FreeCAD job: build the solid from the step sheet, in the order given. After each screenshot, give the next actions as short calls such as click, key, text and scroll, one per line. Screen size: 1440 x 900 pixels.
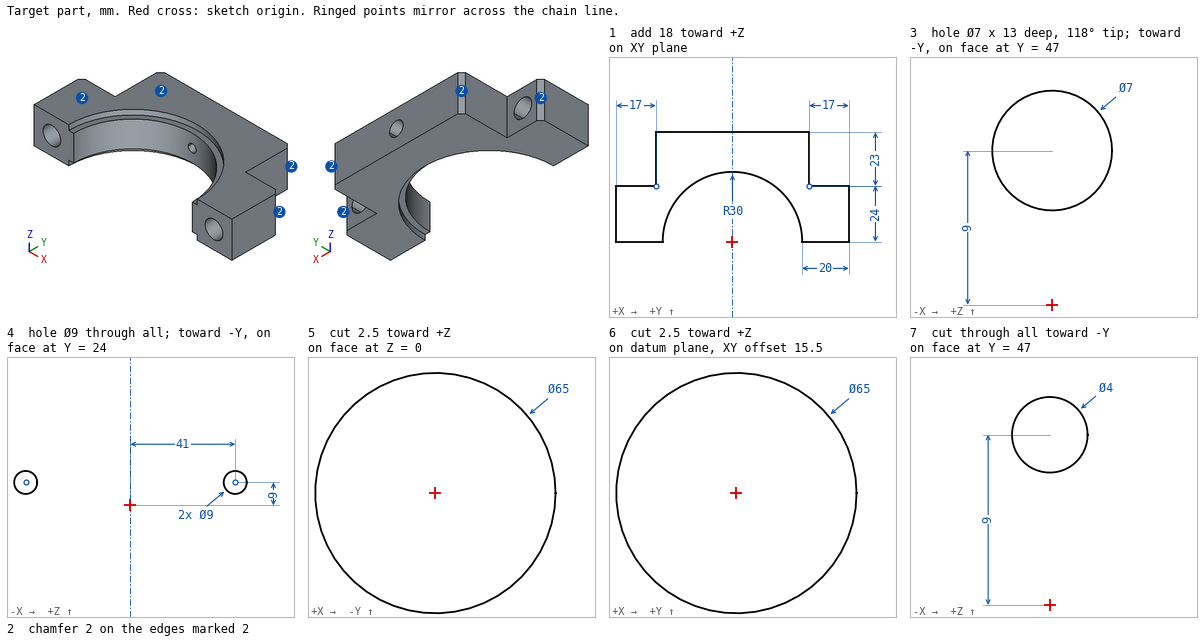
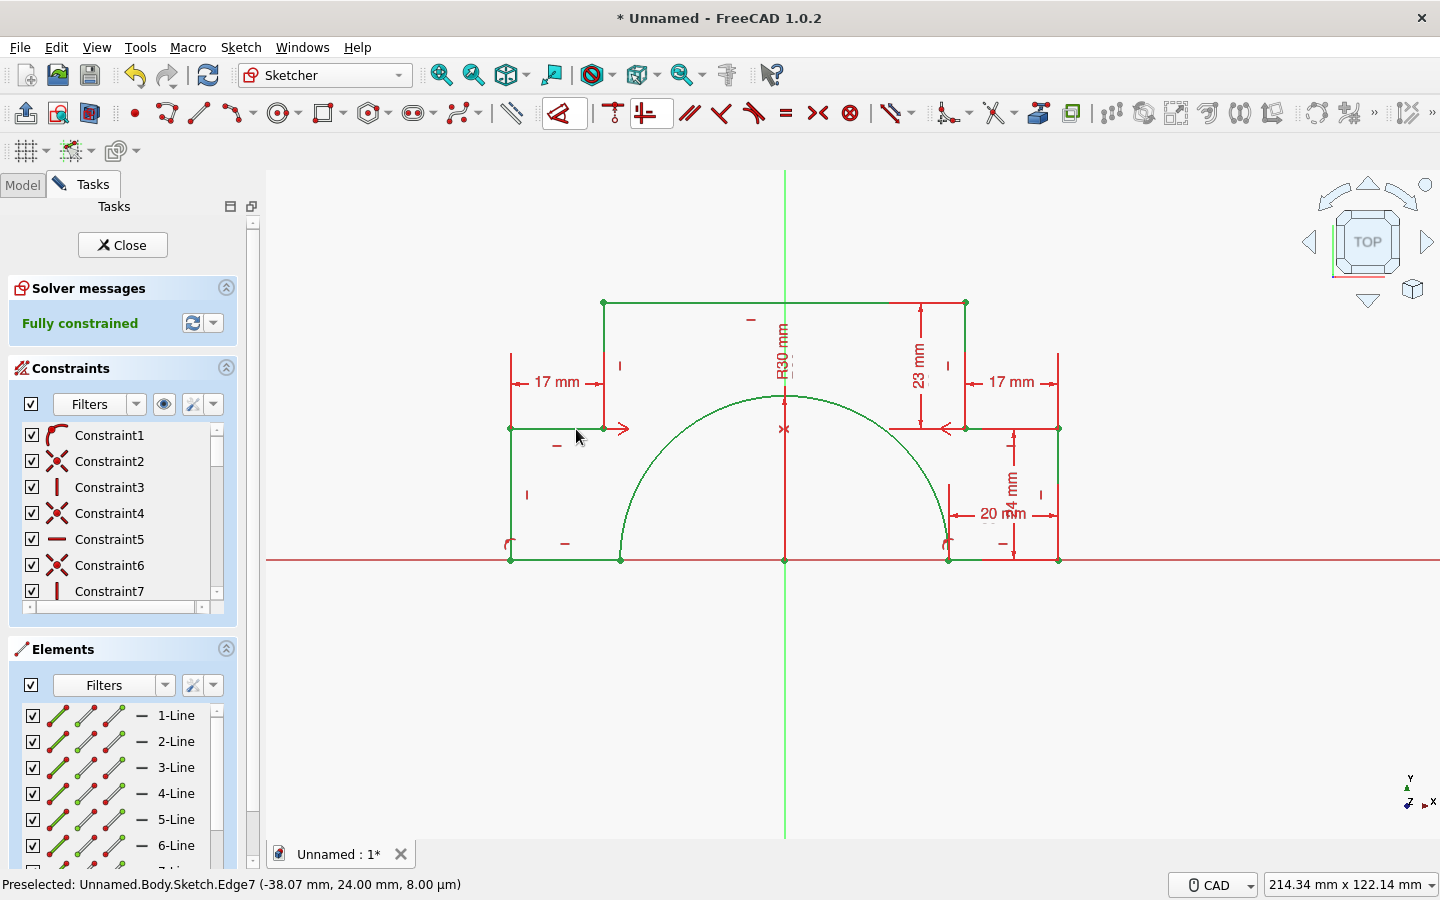
click(123, 245)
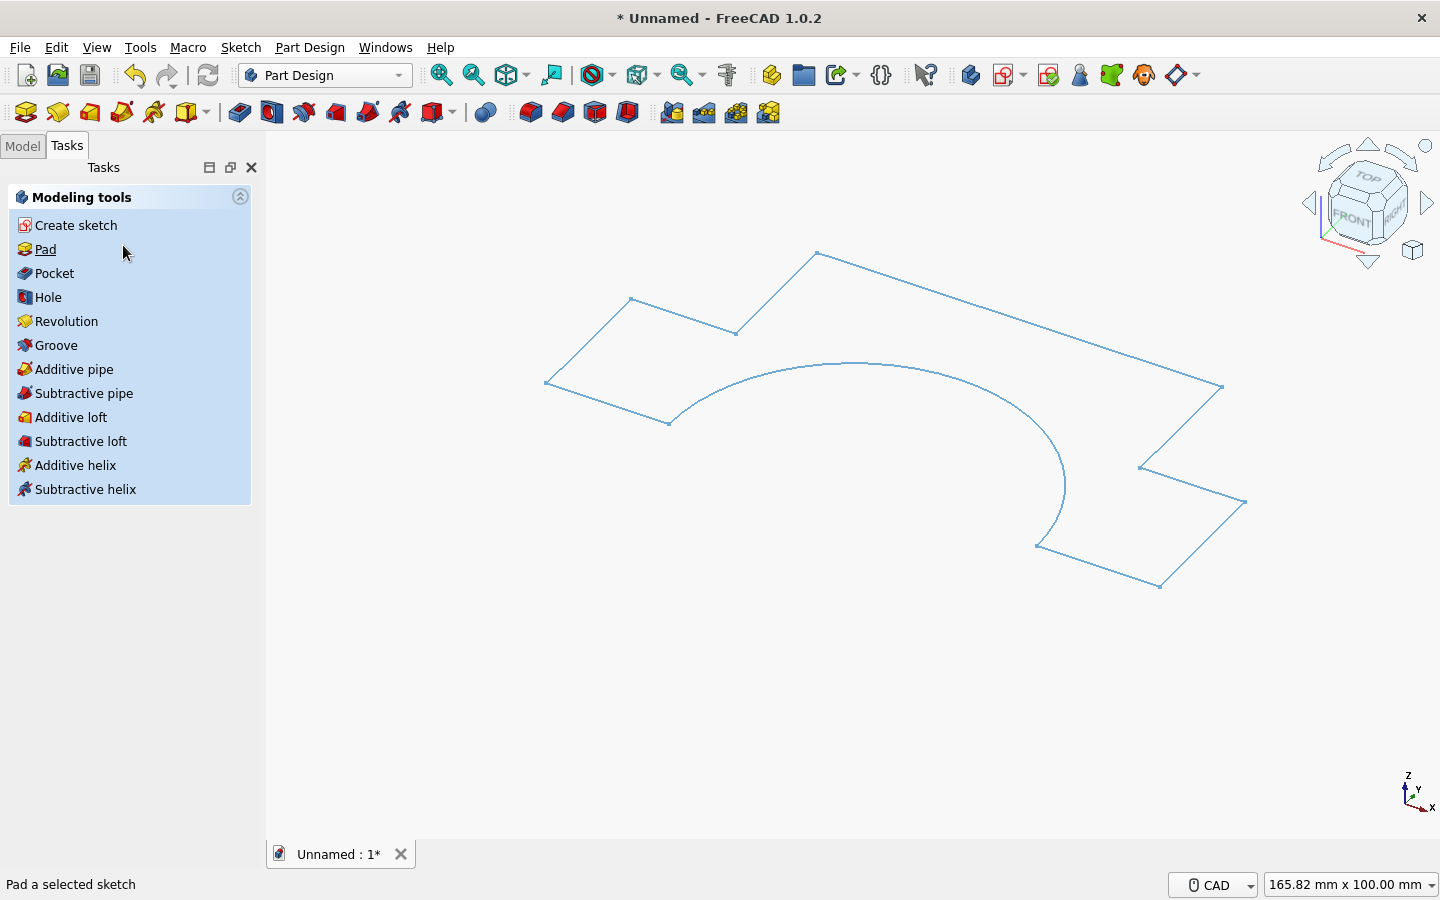
click(26, 112)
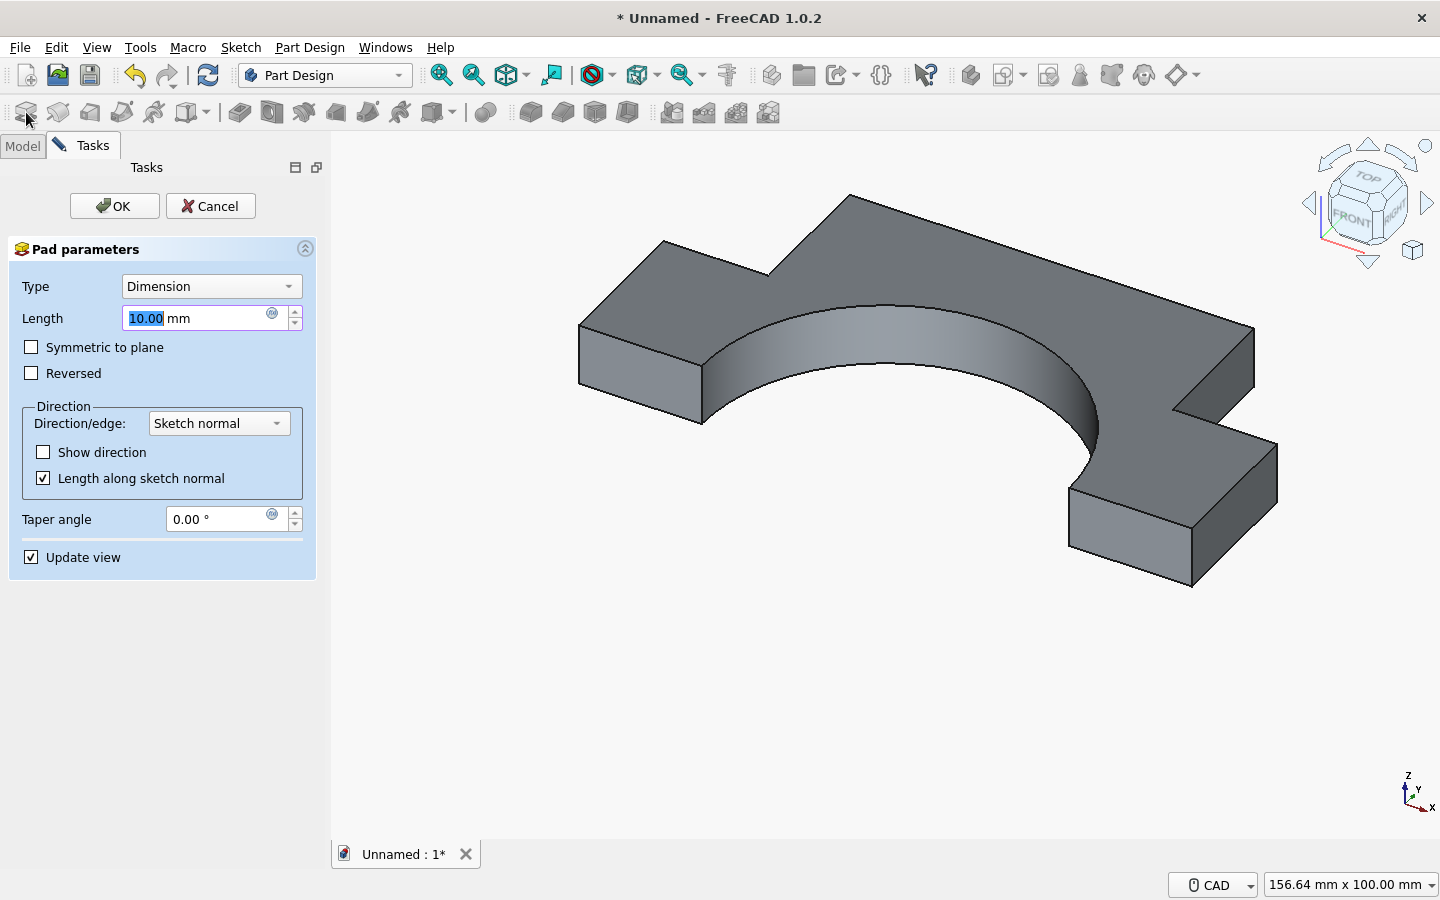
text(18)
key(Tab)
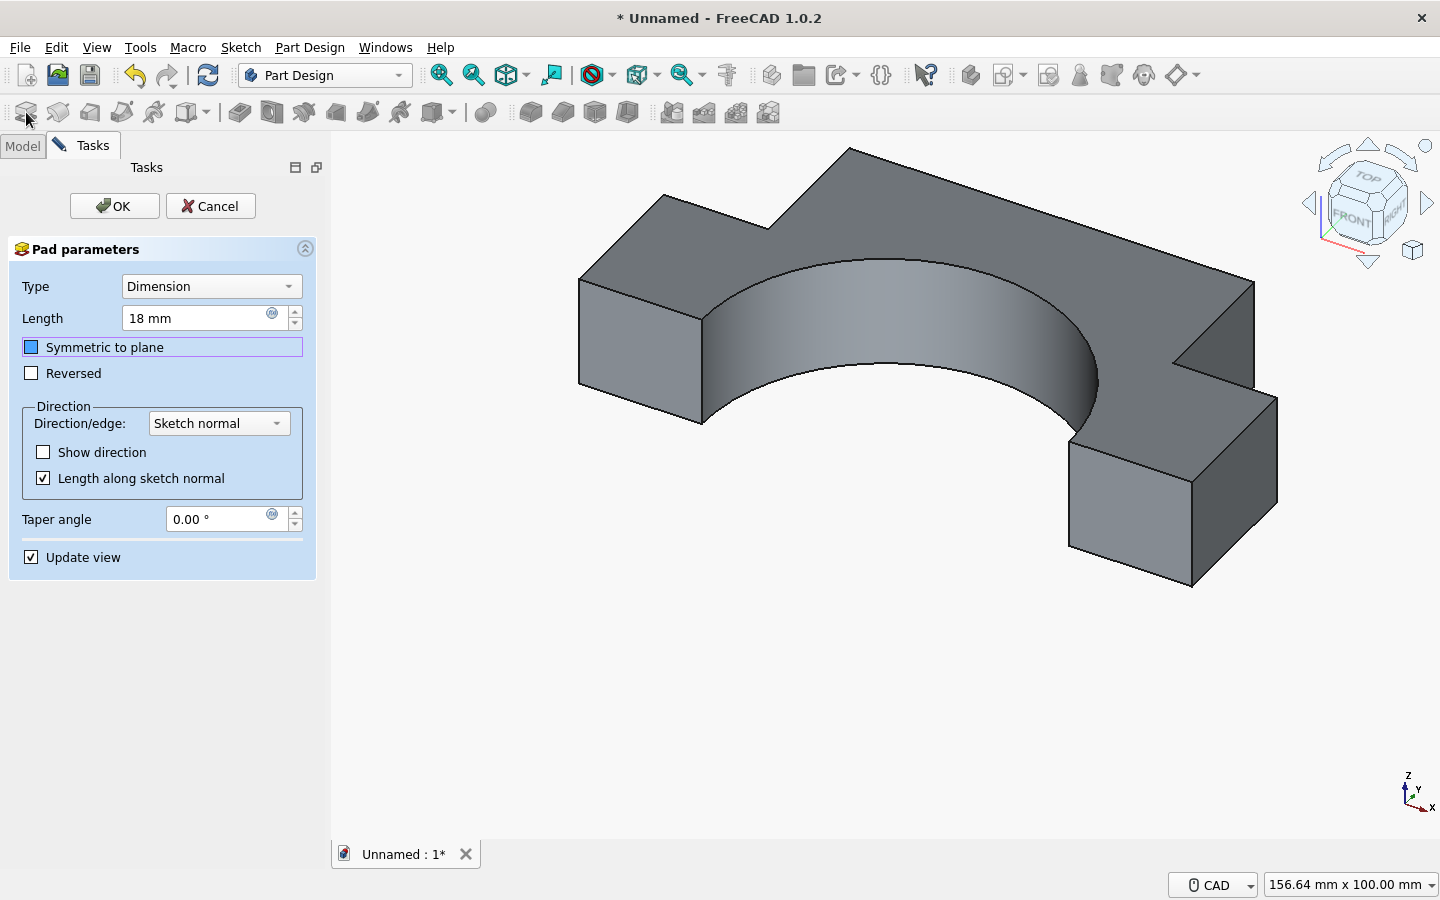
click(115, 206)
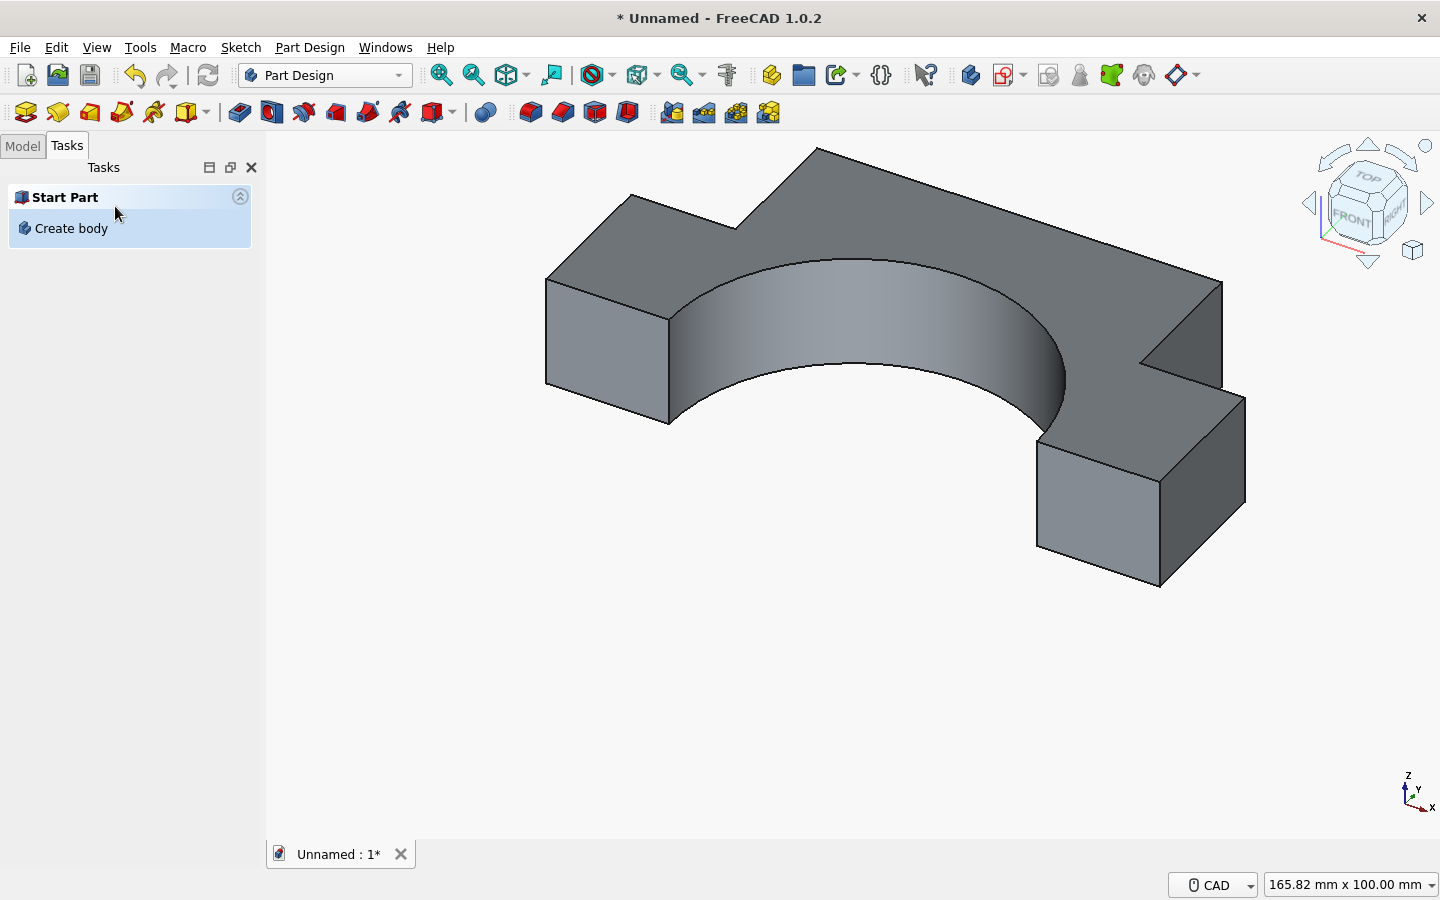
click(442, 76)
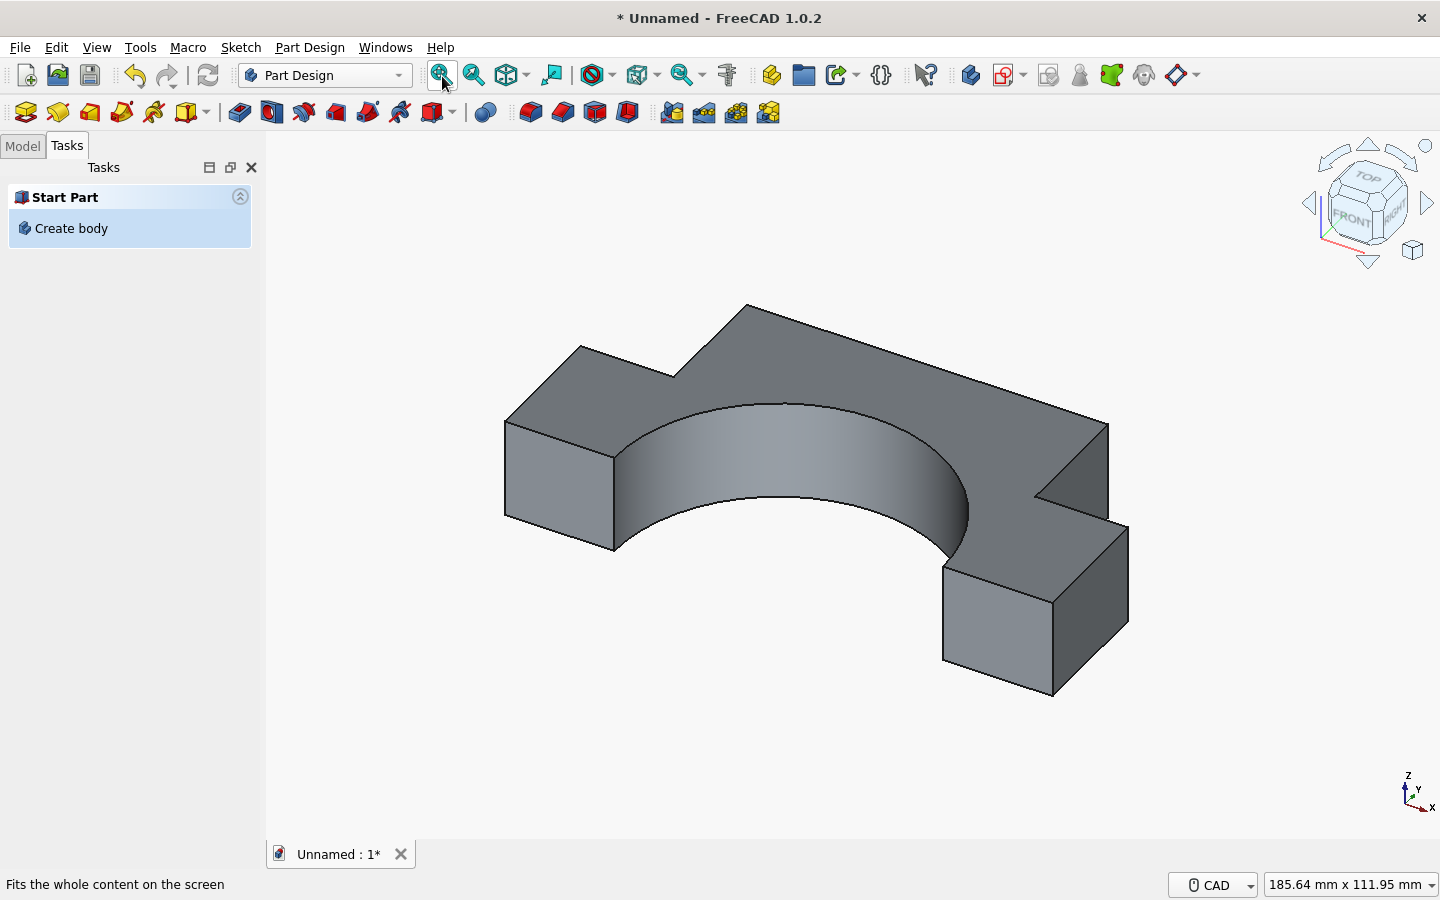
key(0)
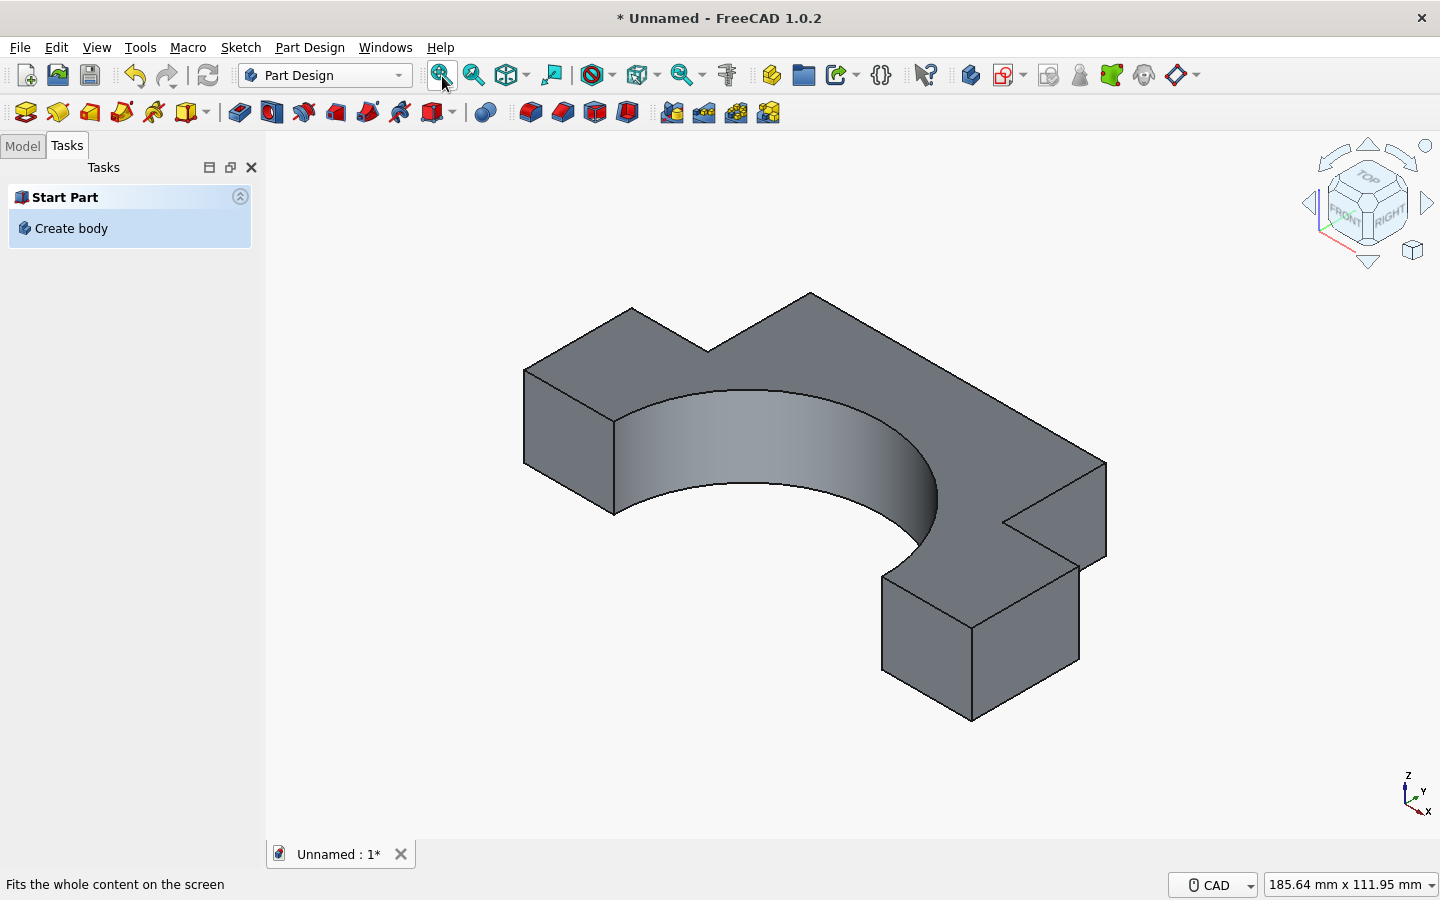
key(2)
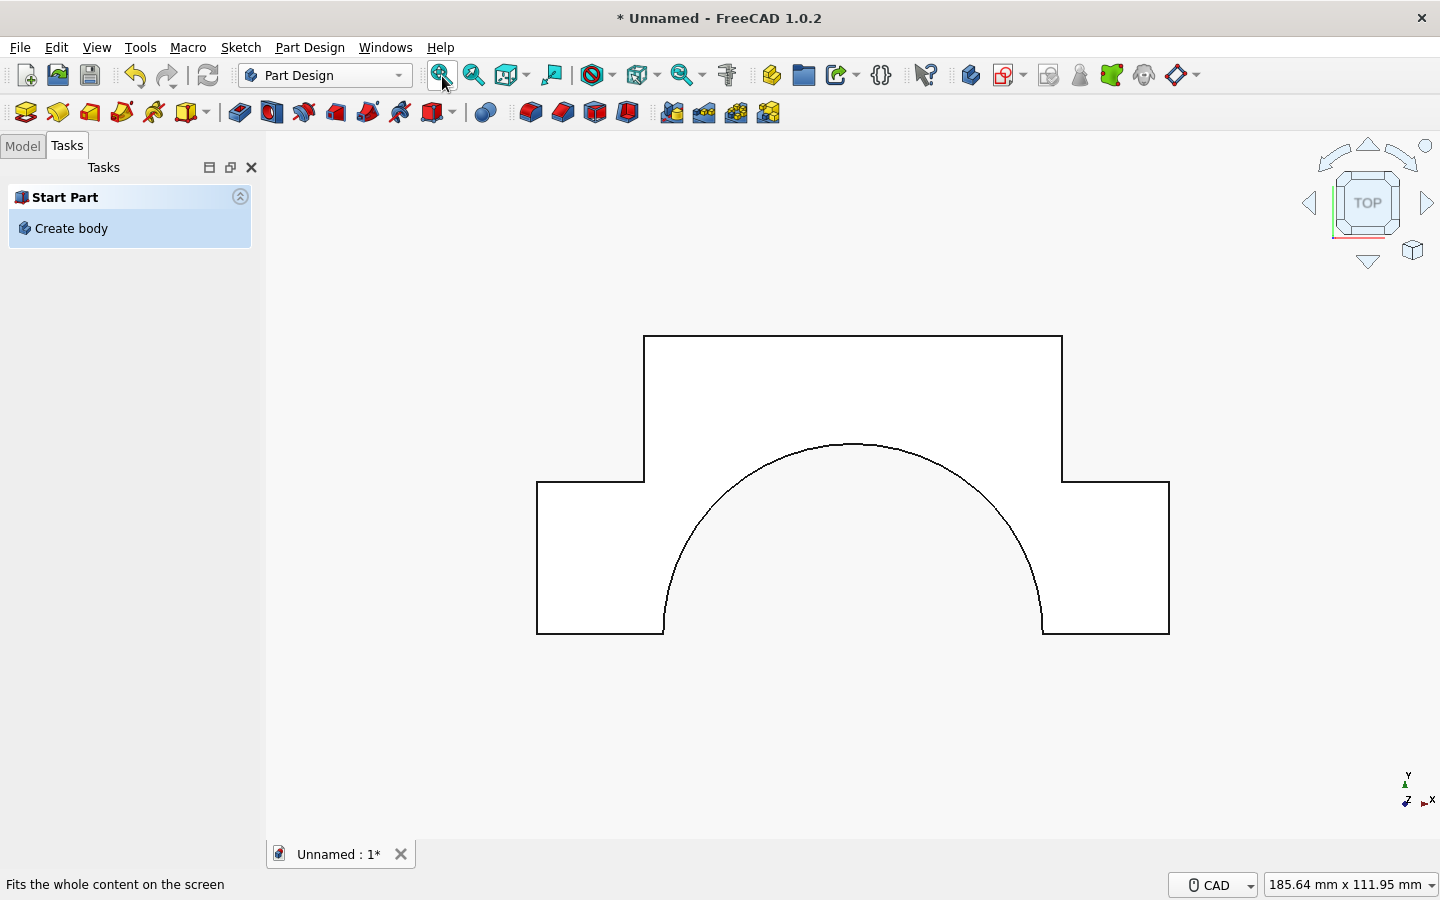
key(1)